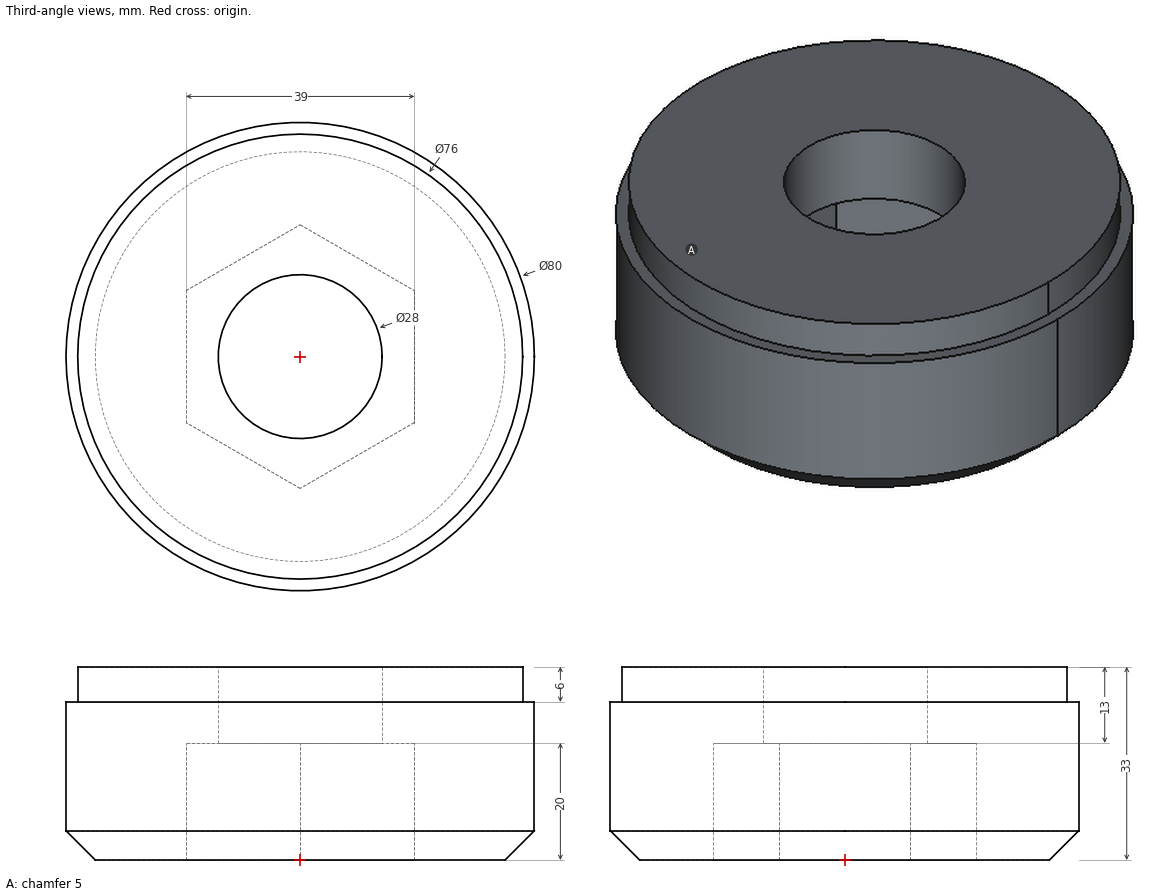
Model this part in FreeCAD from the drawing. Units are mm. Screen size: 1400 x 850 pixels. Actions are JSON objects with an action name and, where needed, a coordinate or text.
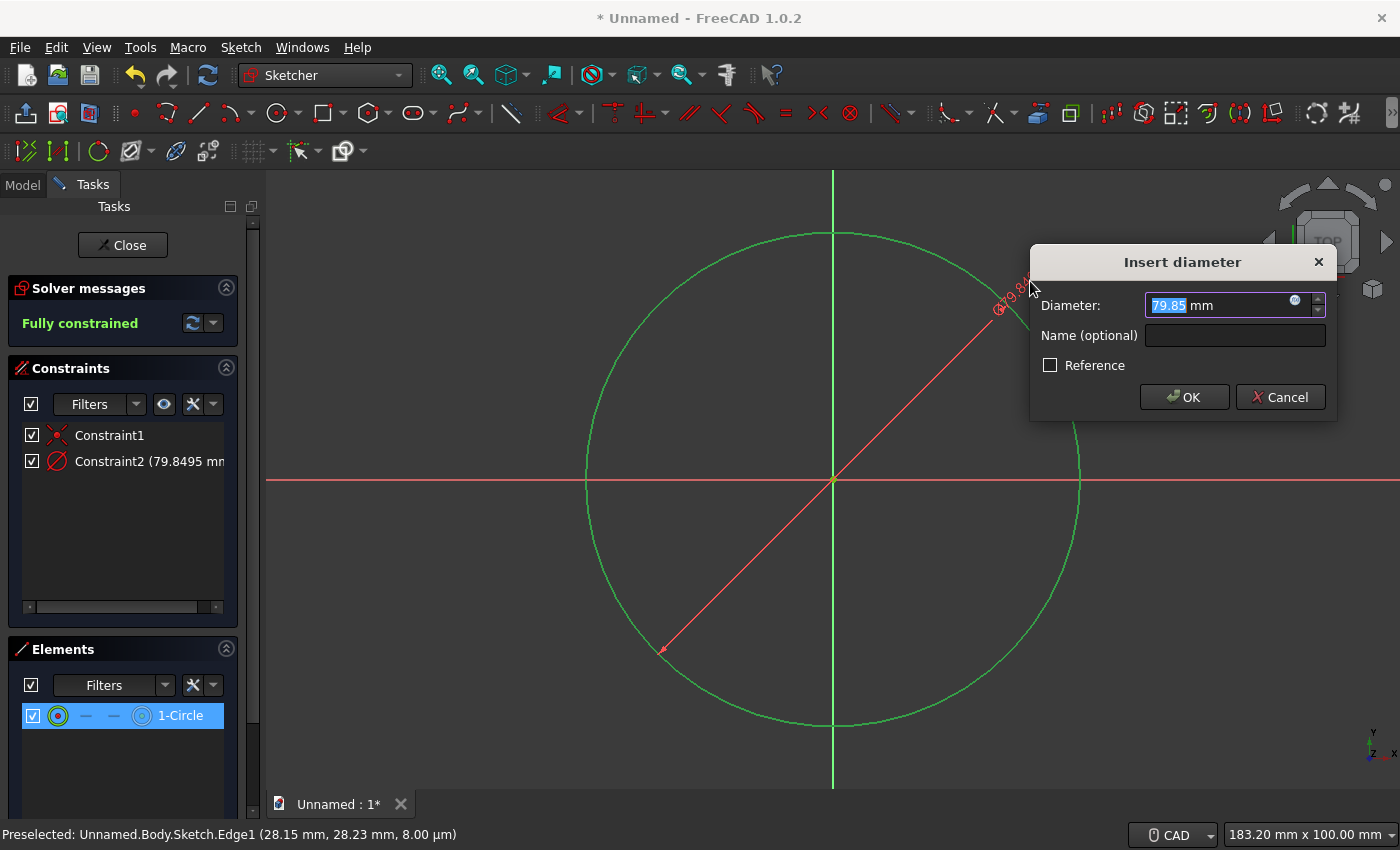
{"action": "type", "text": "80"}
{"action": "key", "text": "Return"}
{"action": "key", "text": "Escape"}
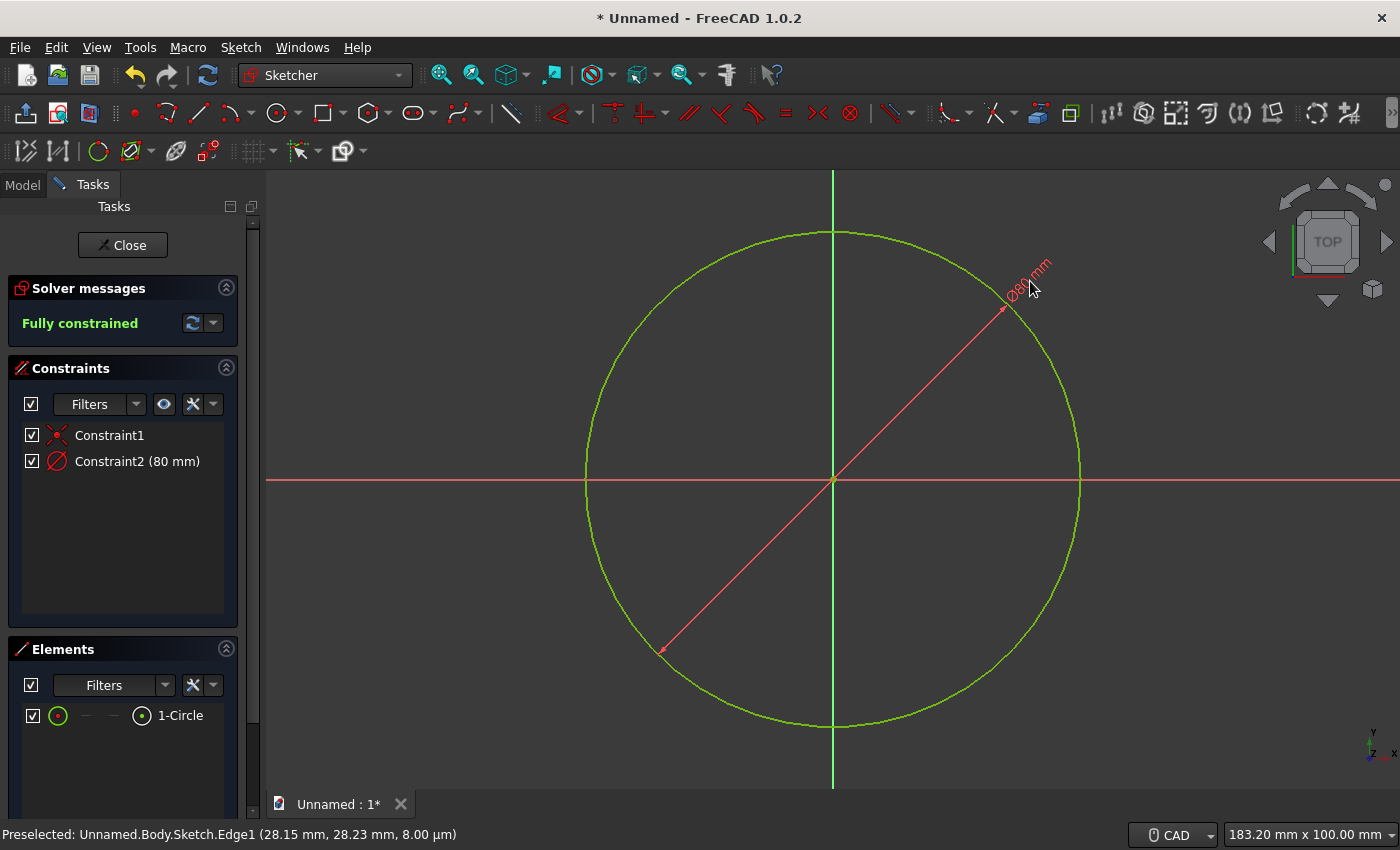
{"action": "left_click", "coordinate": [123, 245]}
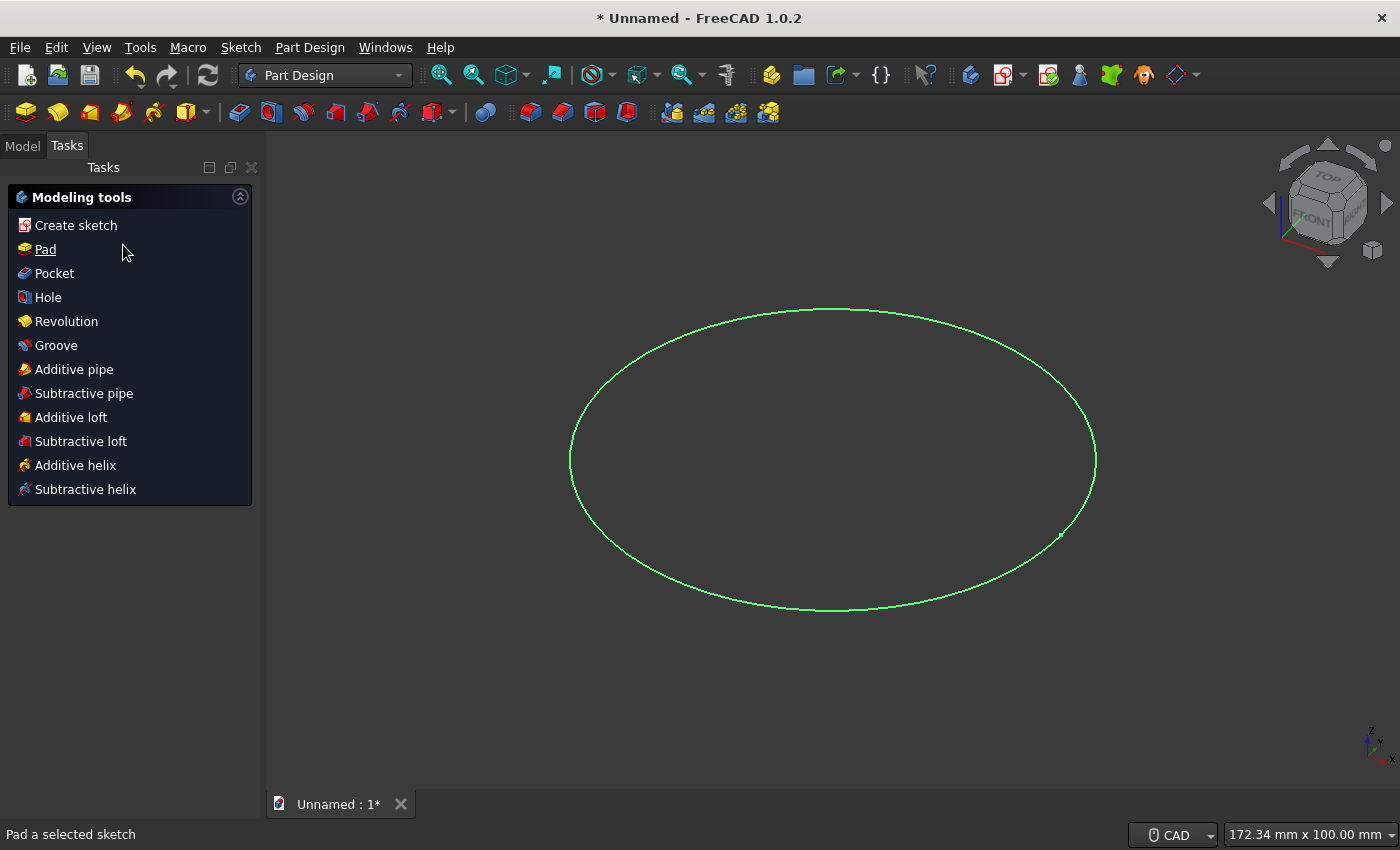
{"action": "left_click", "coordinate": [26, 112]}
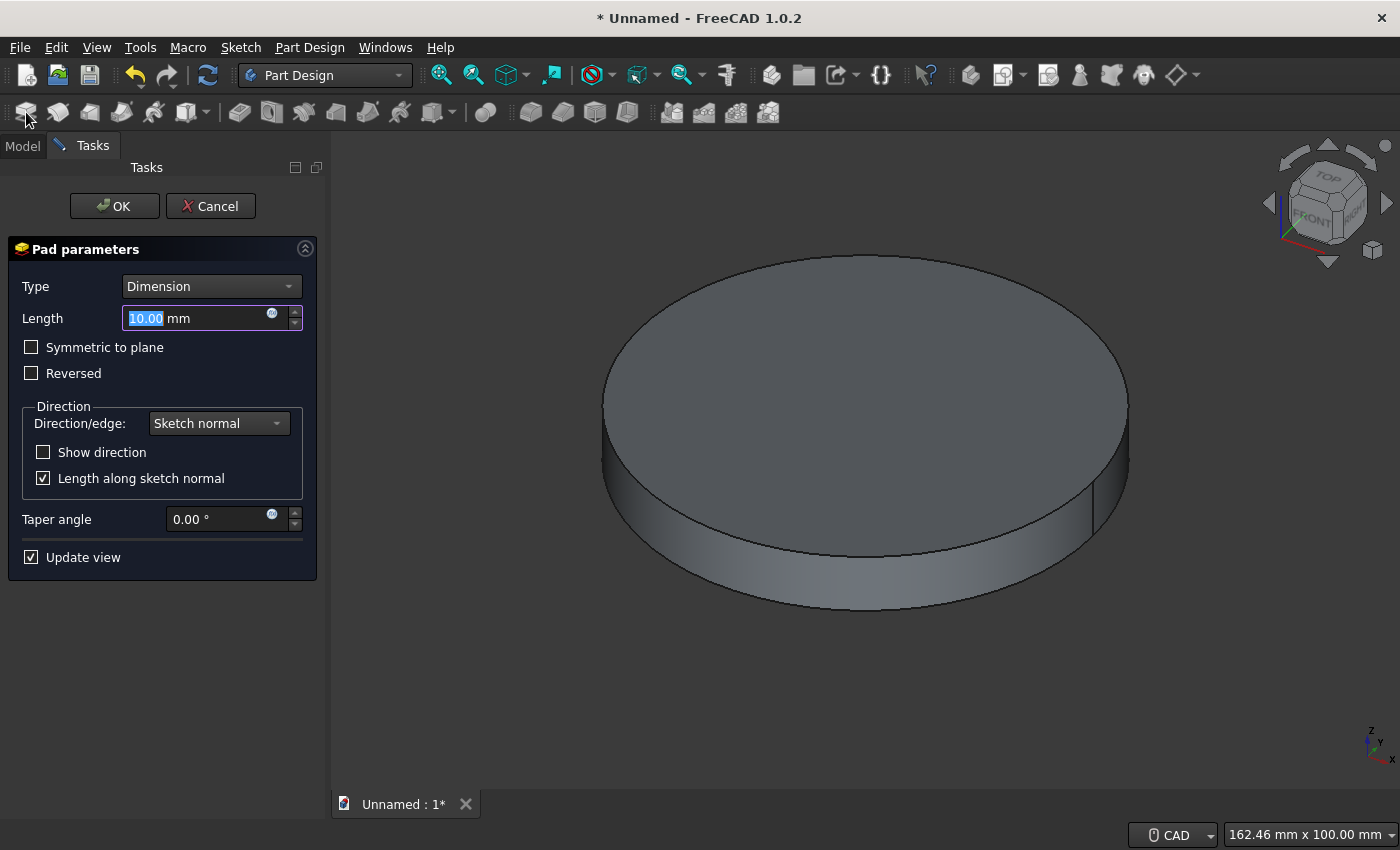
{"action": "type", "text": "33"}
{"action": "key", "text": "Tab"}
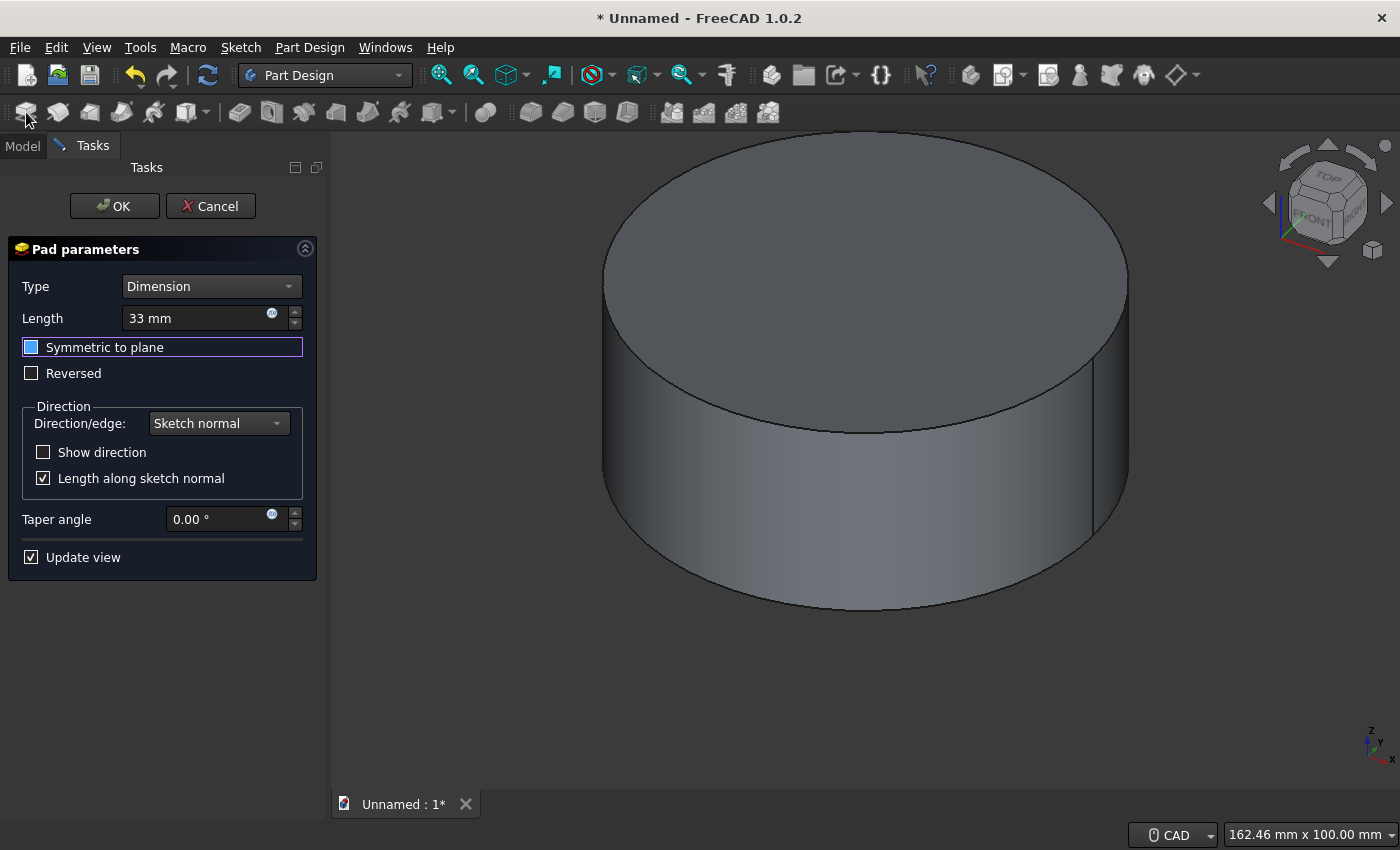
{"action": "left_click", "coordinate": [115, 206]}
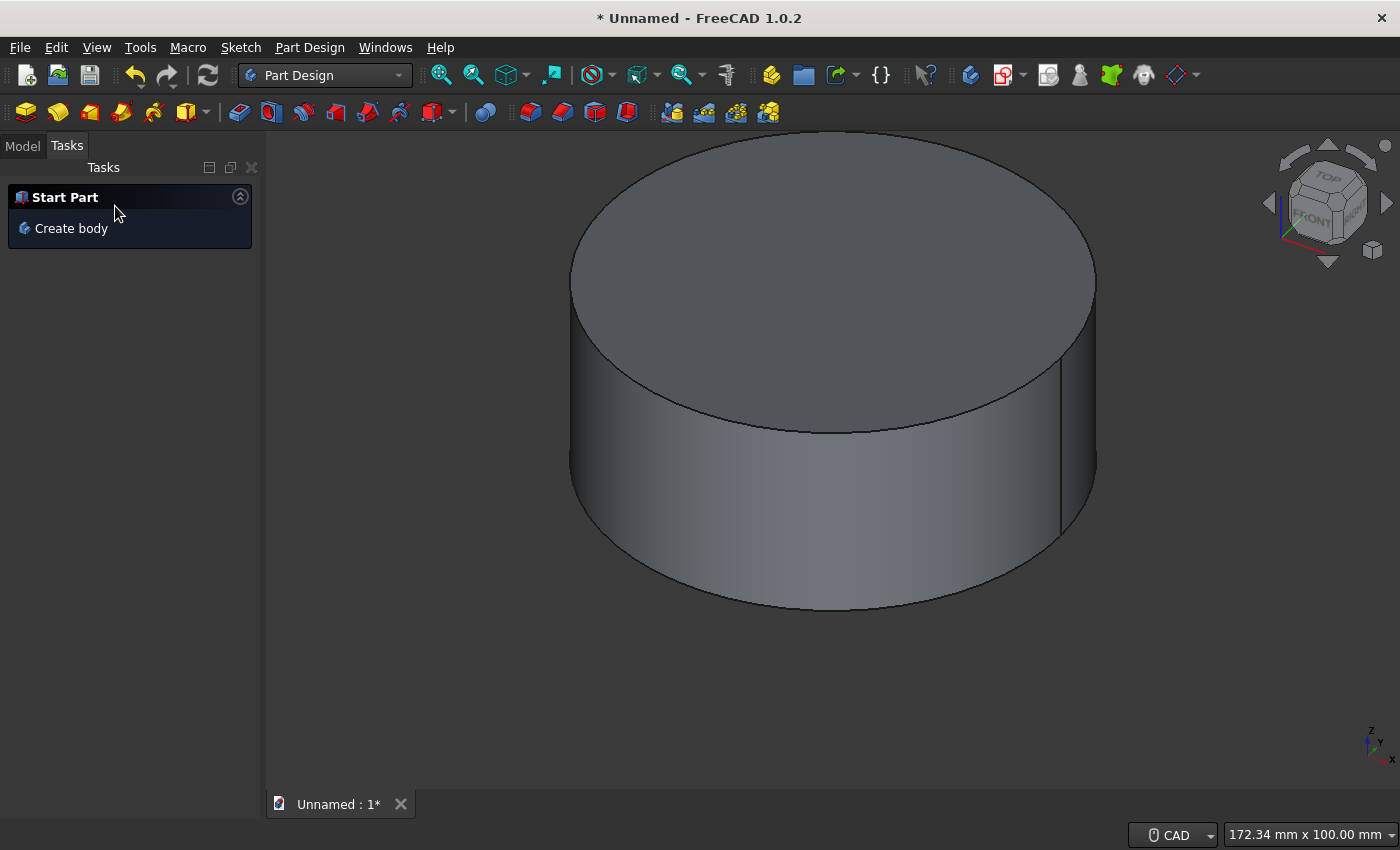
{"action": "left_click", "coordinate": [442, 76]}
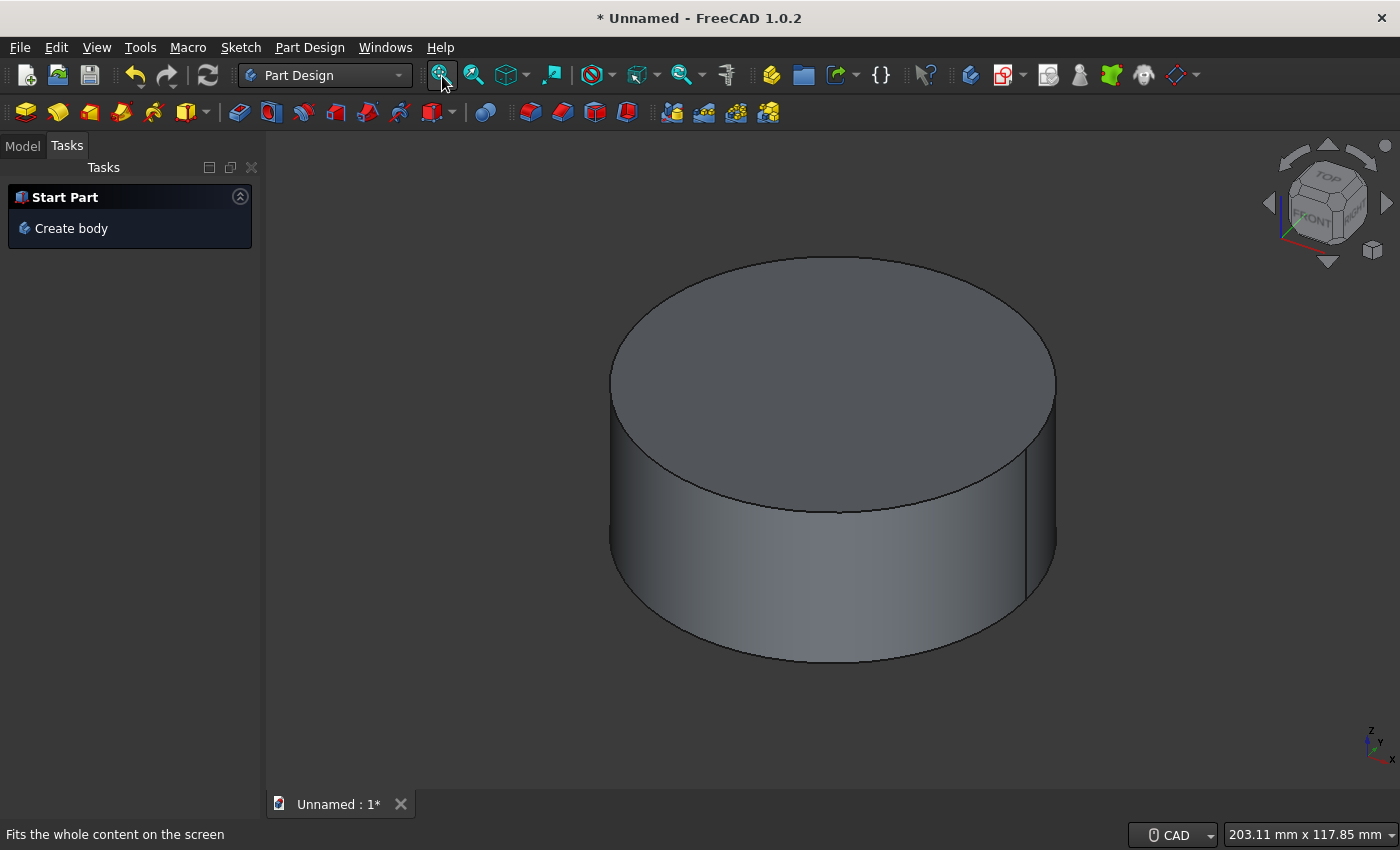
{"action": "left_click", "coordinate": [23, 145]}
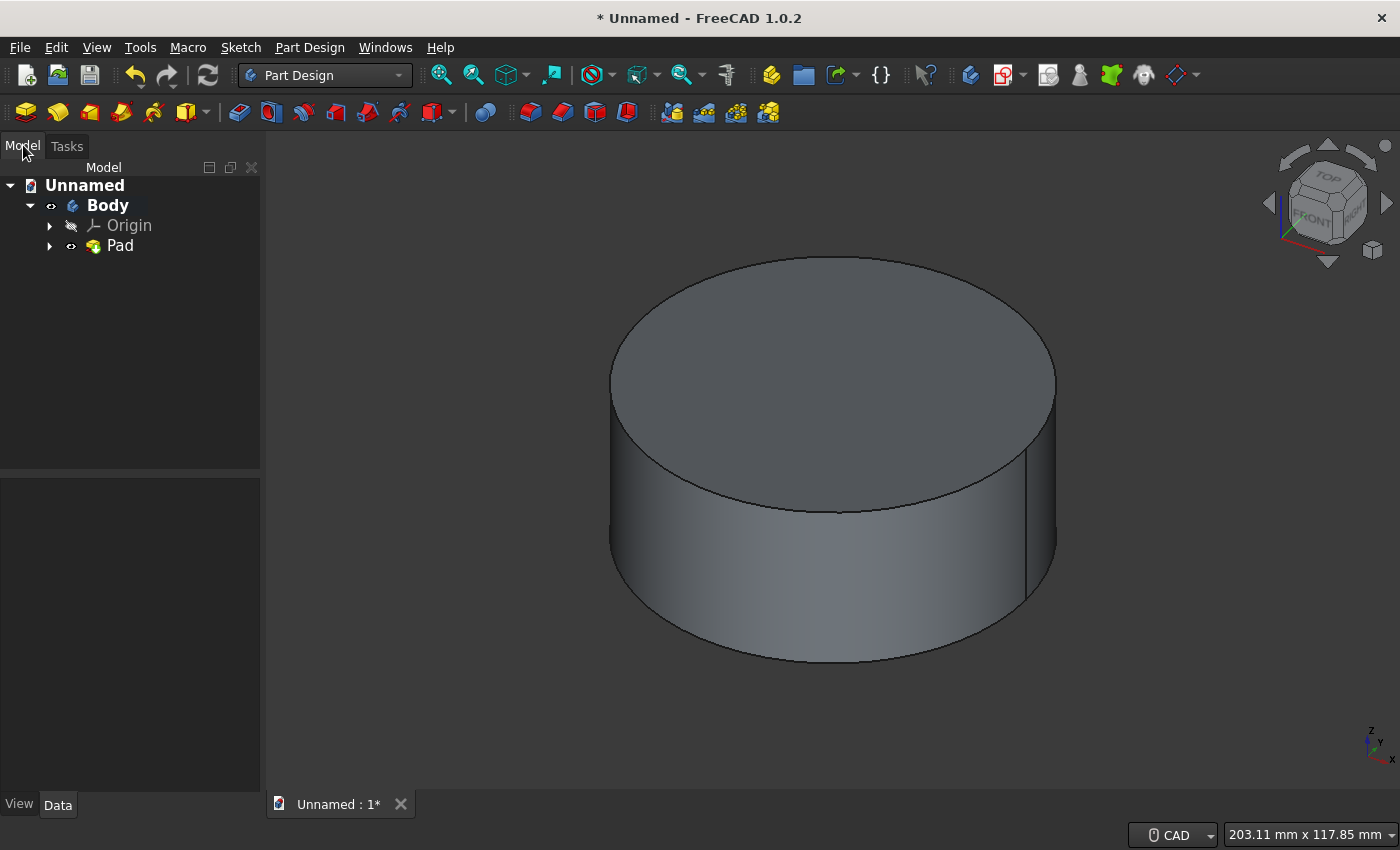
{"action": "left_click", "coordinate": [50, 226]}